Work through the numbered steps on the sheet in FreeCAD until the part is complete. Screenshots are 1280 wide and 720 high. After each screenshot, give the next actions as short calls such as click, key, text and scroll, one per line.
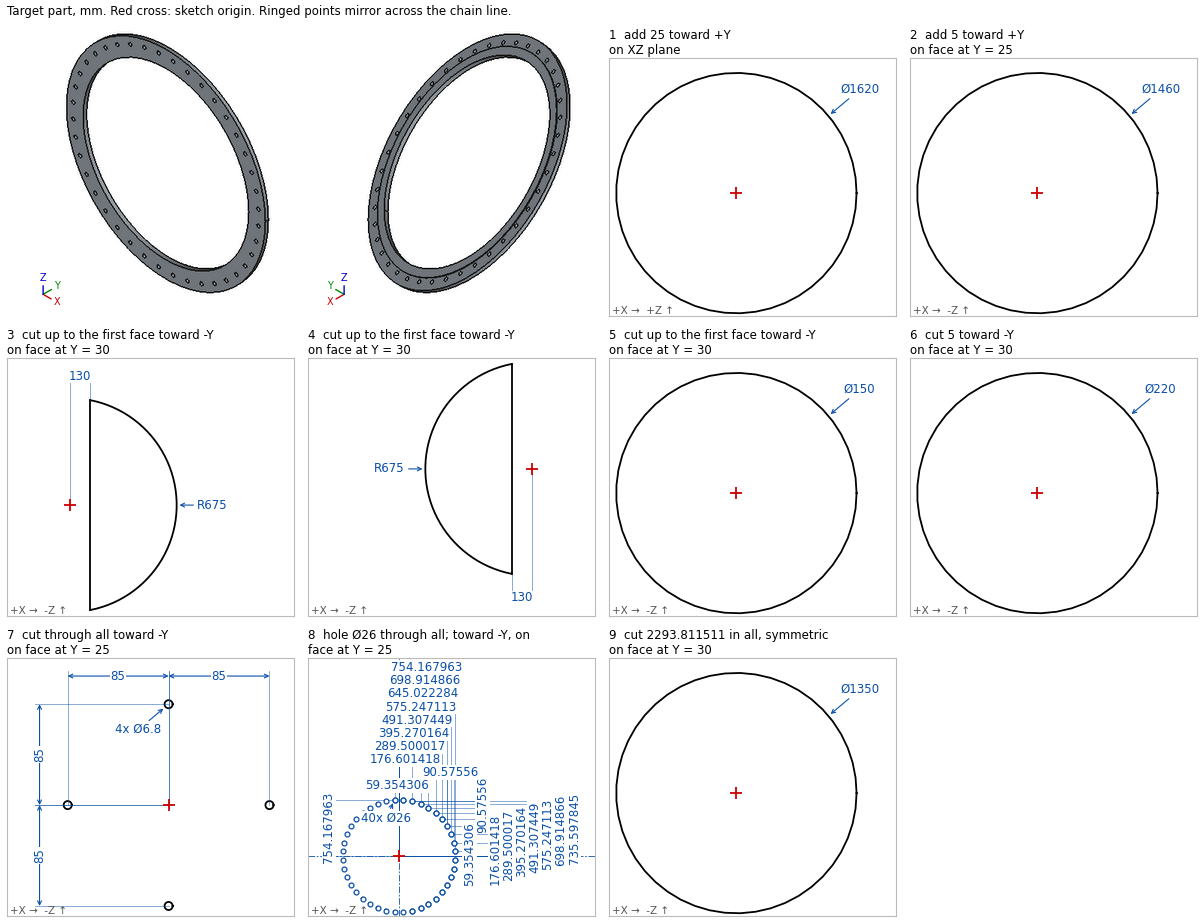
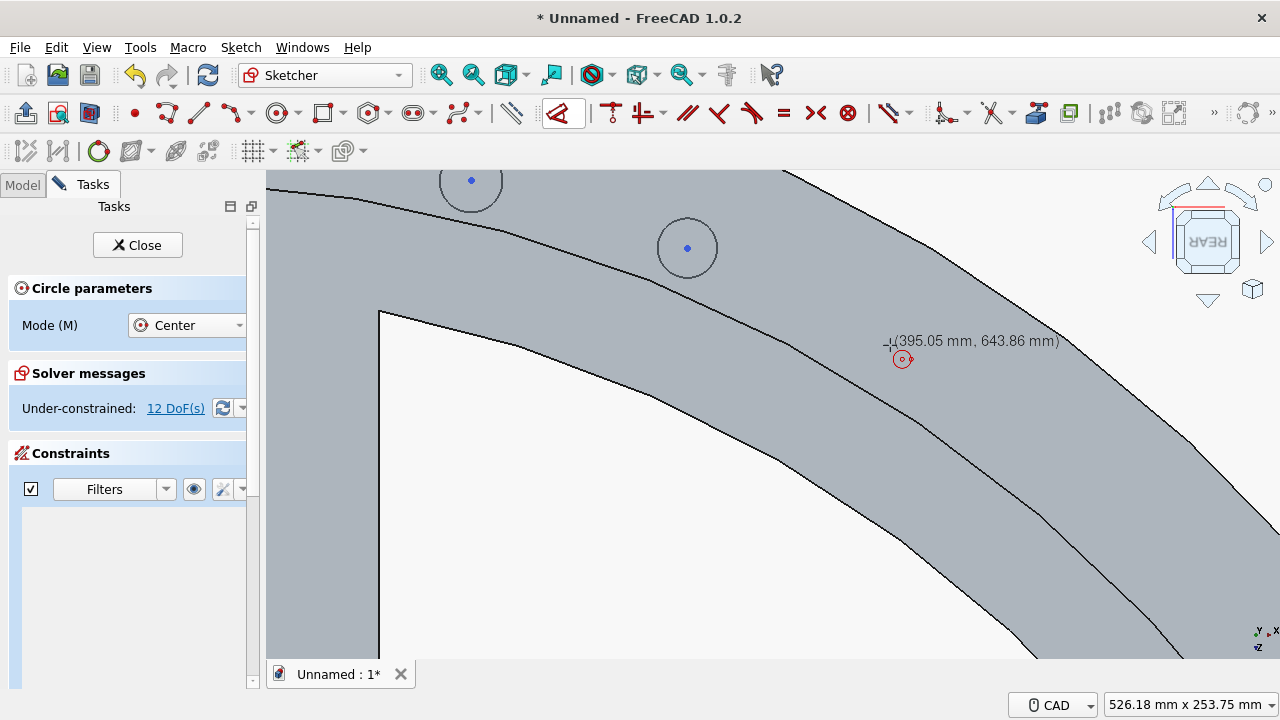
scroll(776, 268, down, 11)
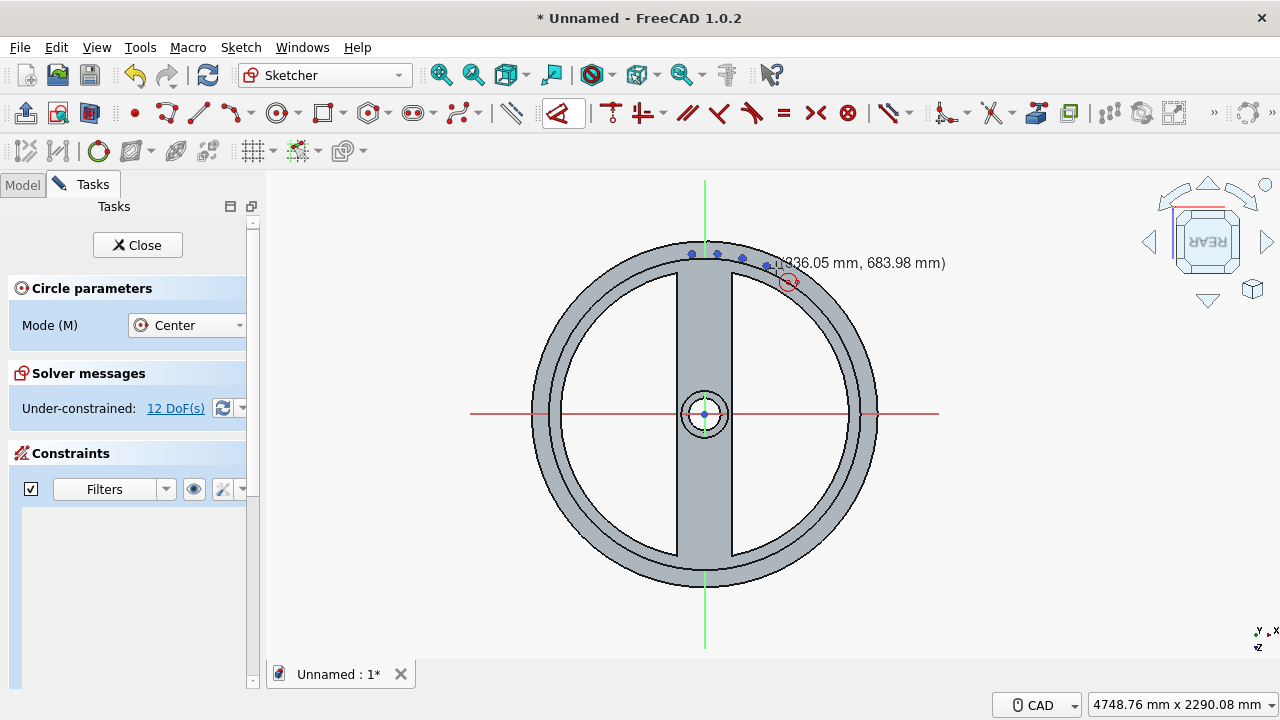
click(789, 277)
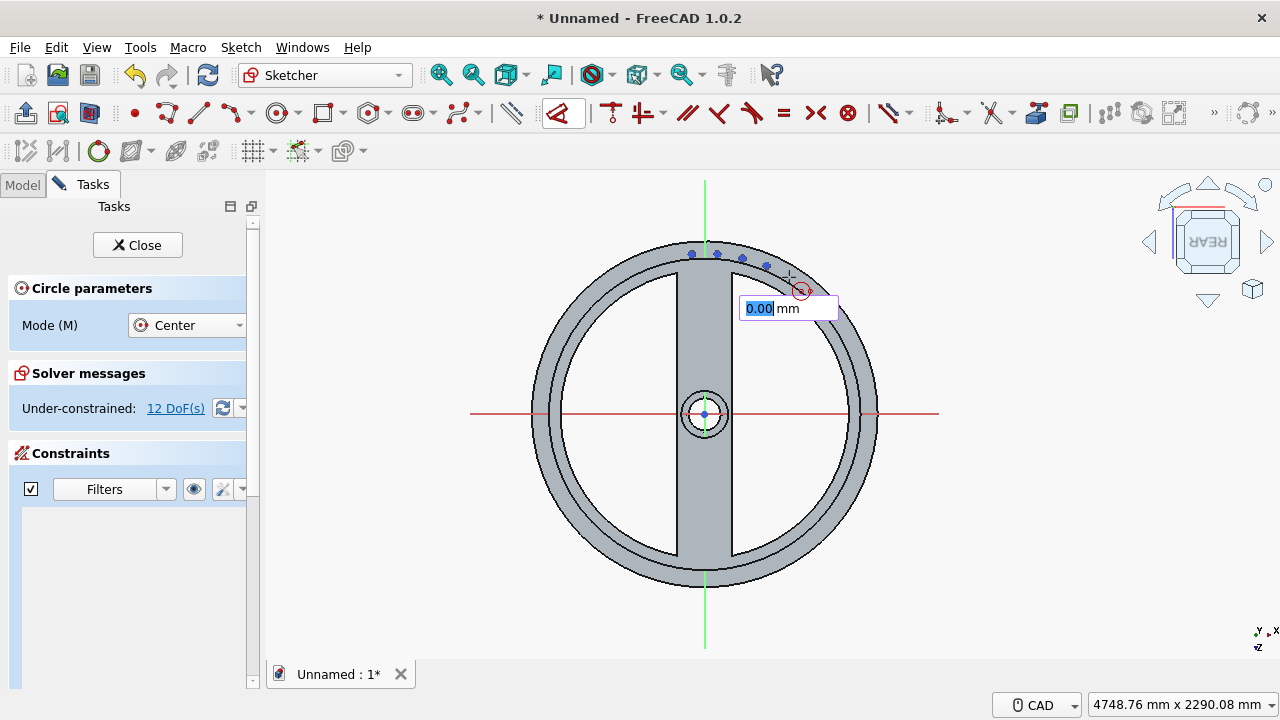
scroll(791, 275, up, 9)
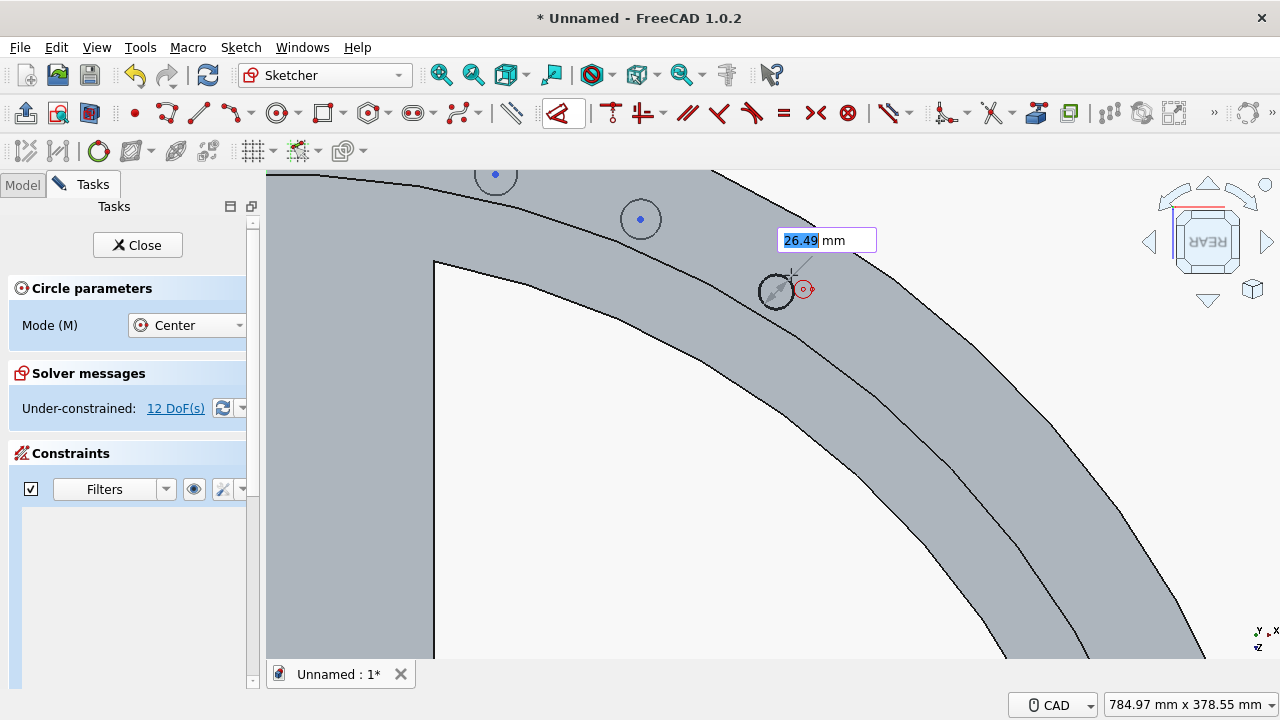
click(789, 272)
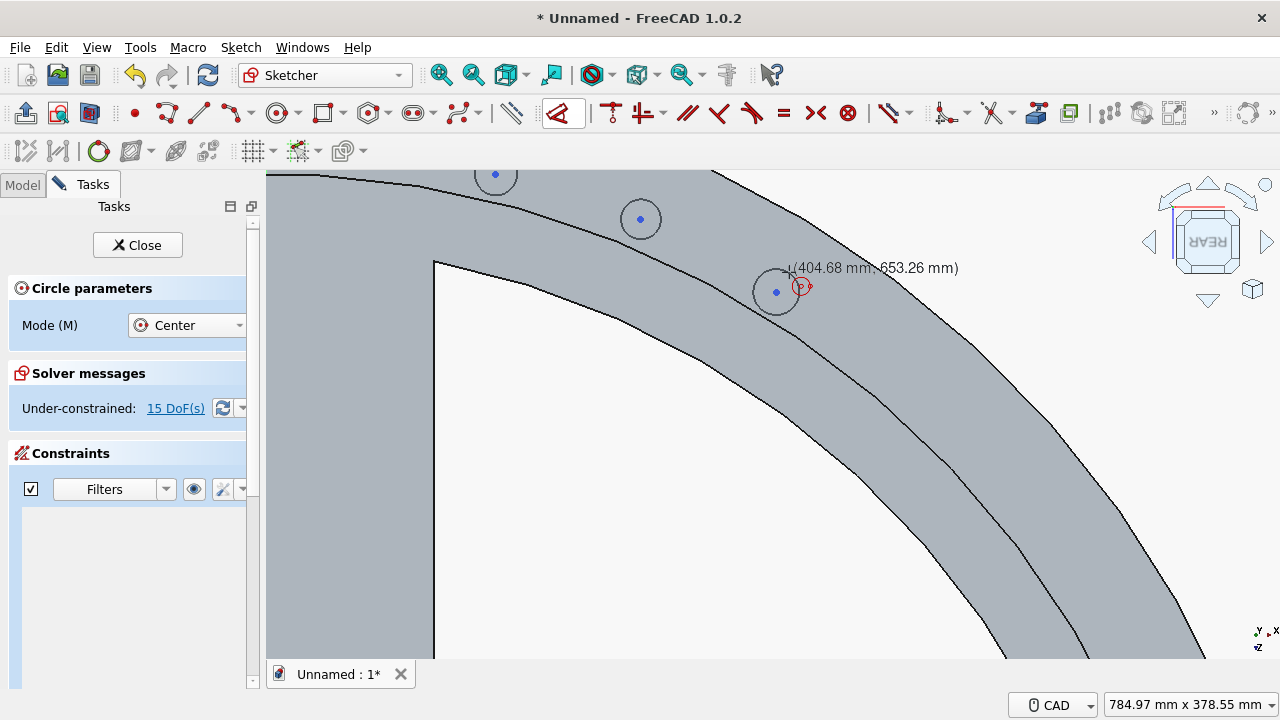
scroll(901, 374, up, 2)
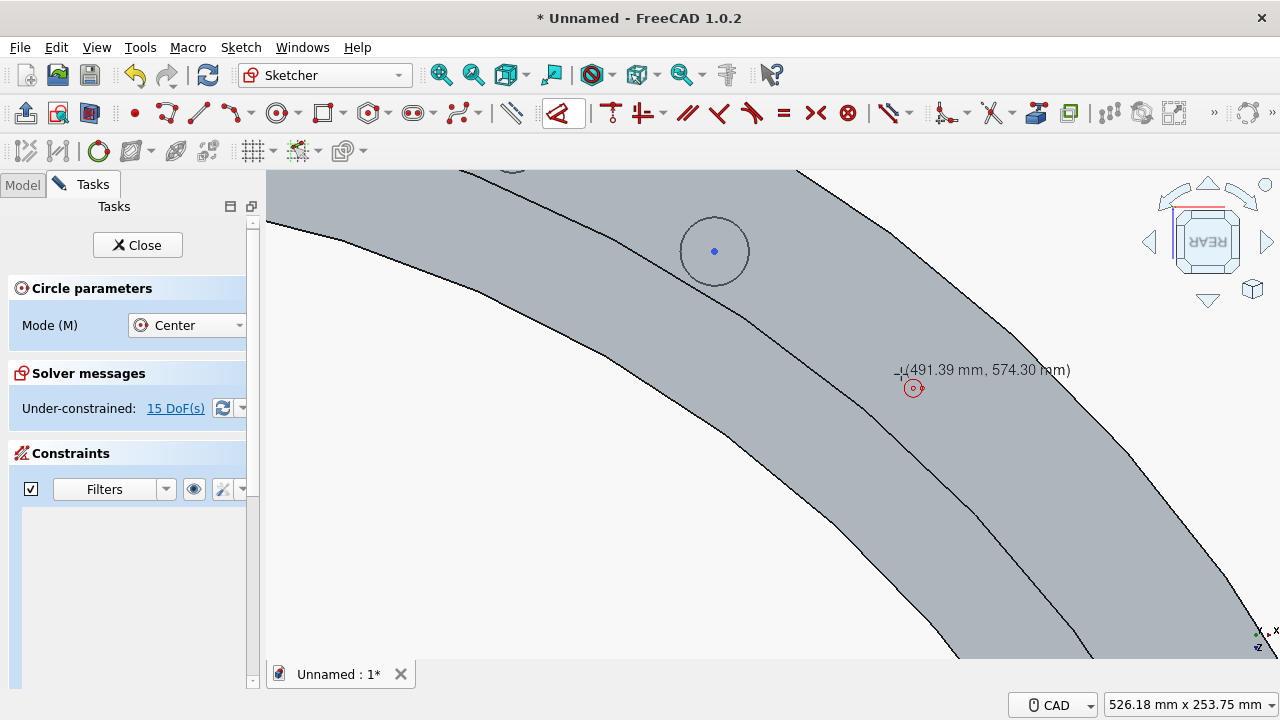
scroll(798, 281, down, 11)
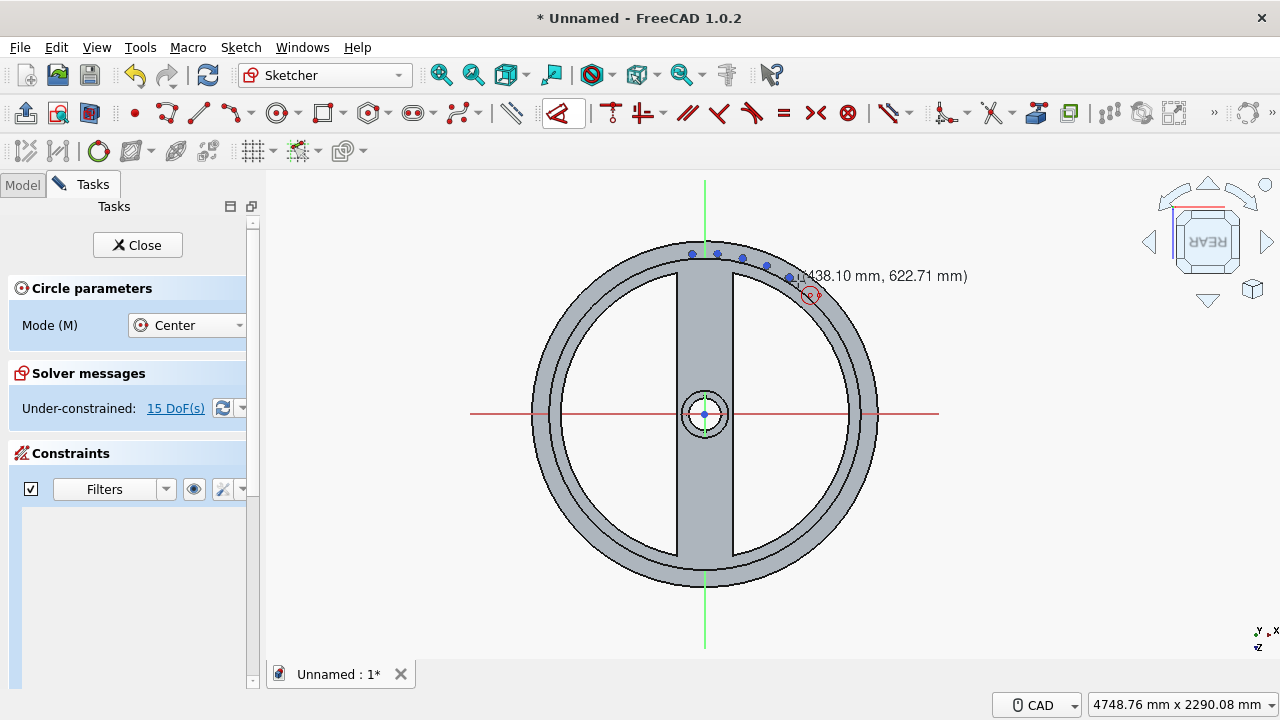
click(810, 291)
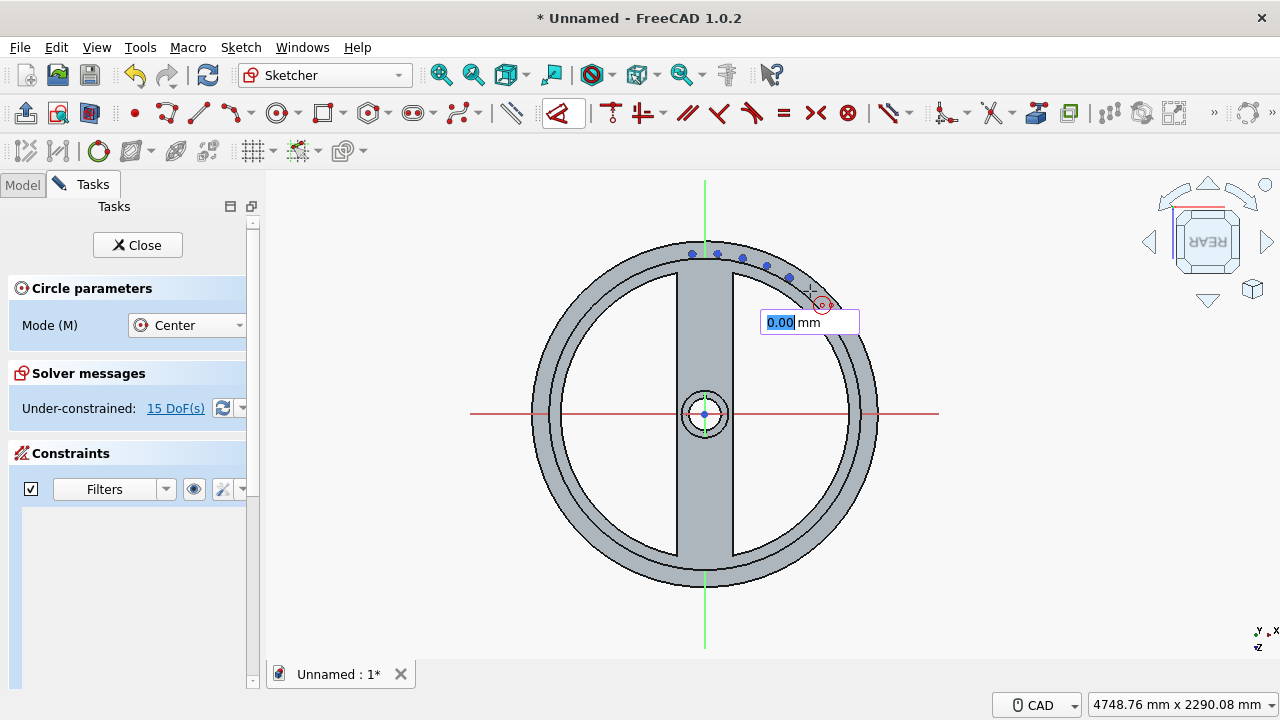
scroll(812, 289, up, 9)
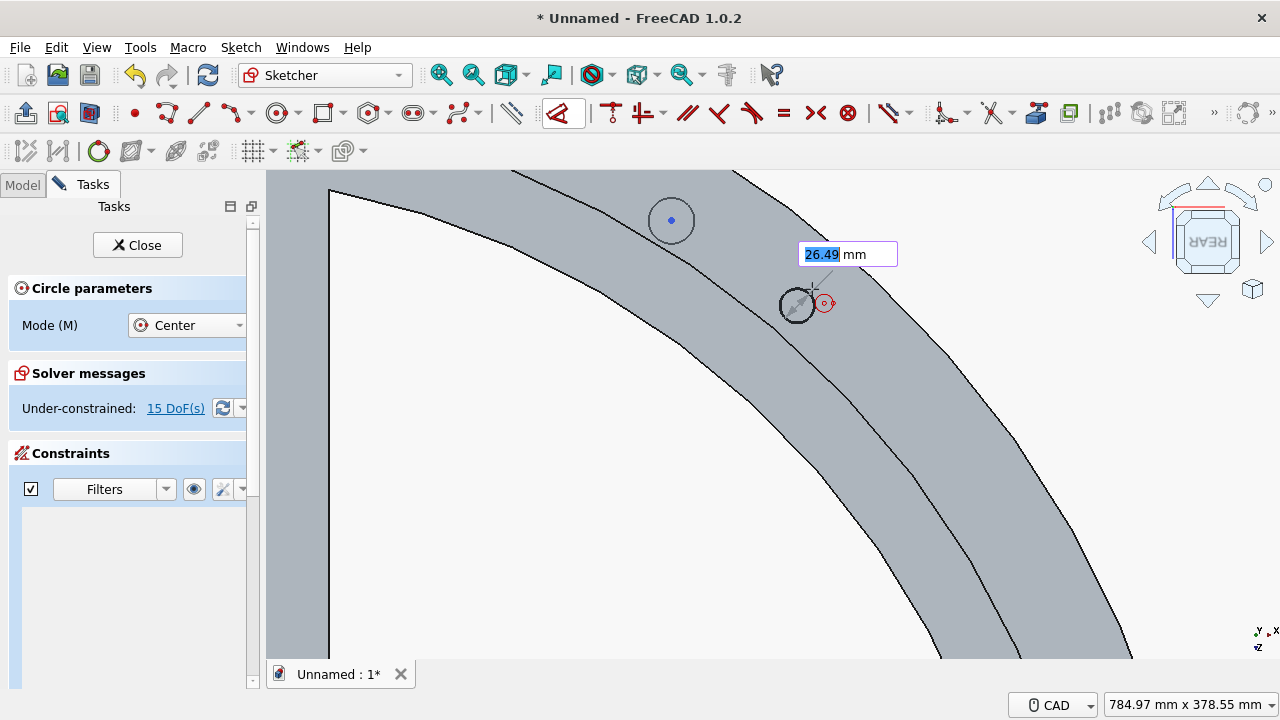
click(808, 291)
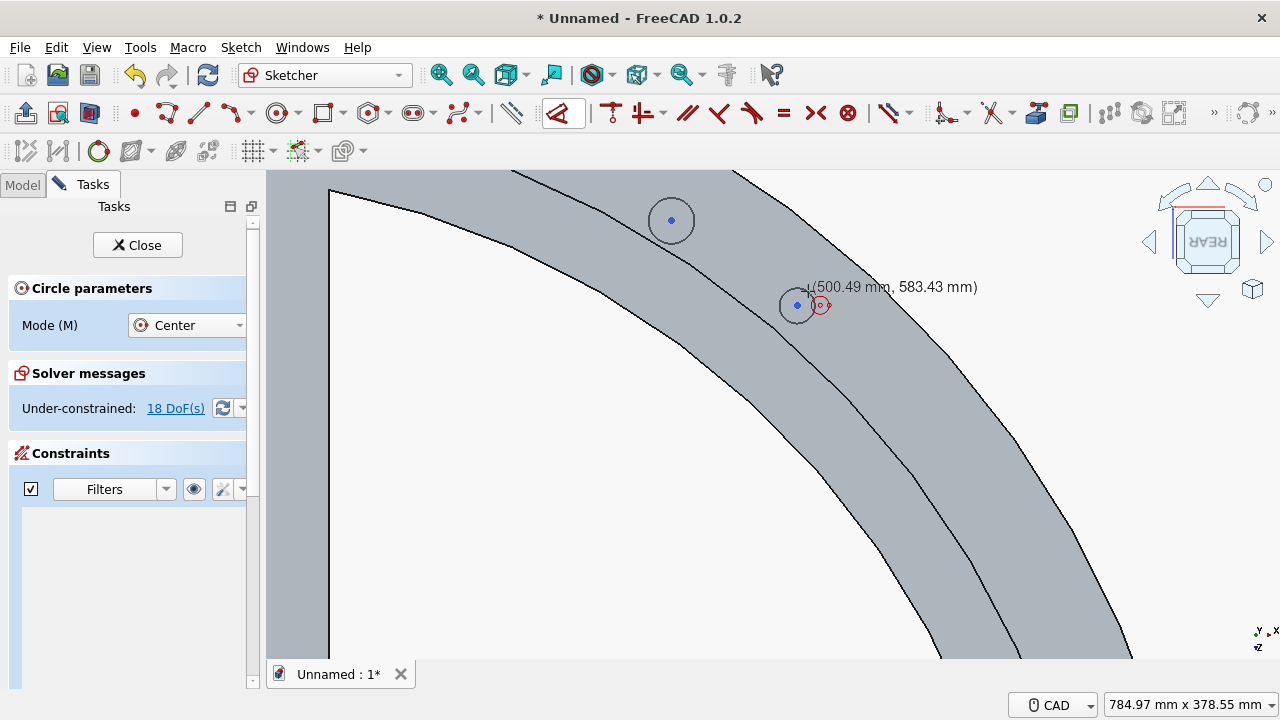
scroll(905, 411, up, 2)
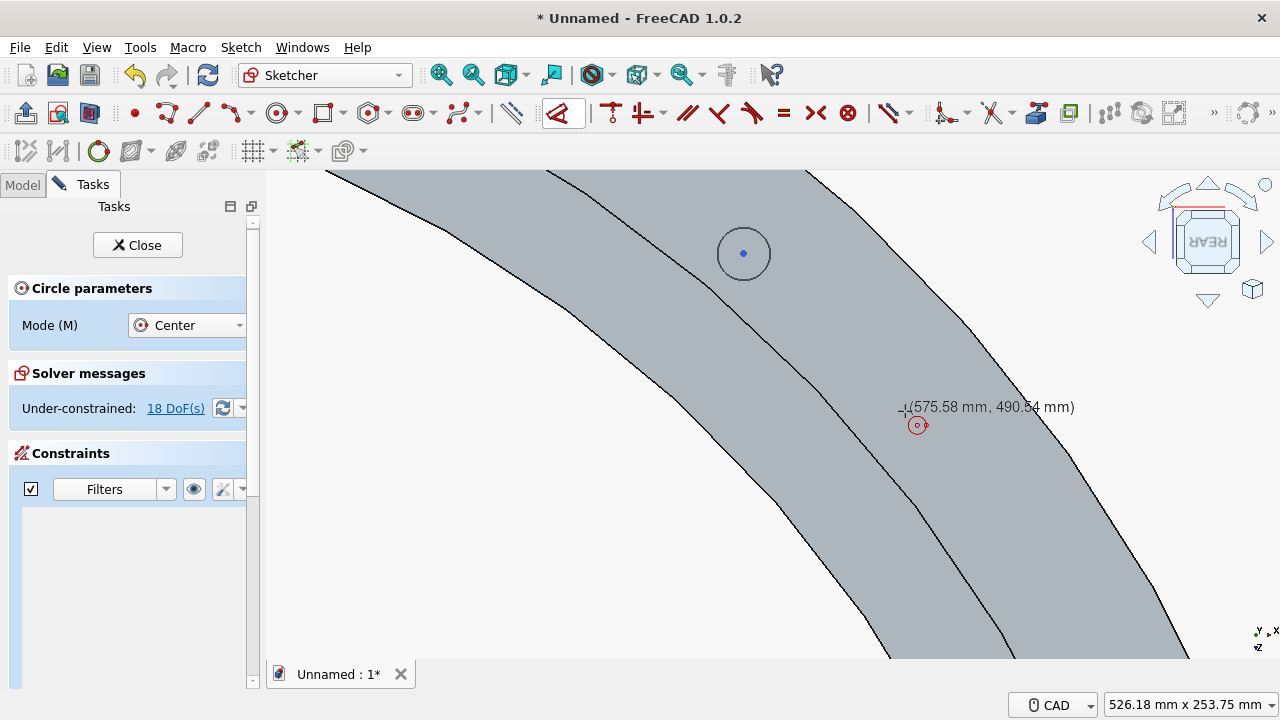
scroll(818, 297, down, 11)